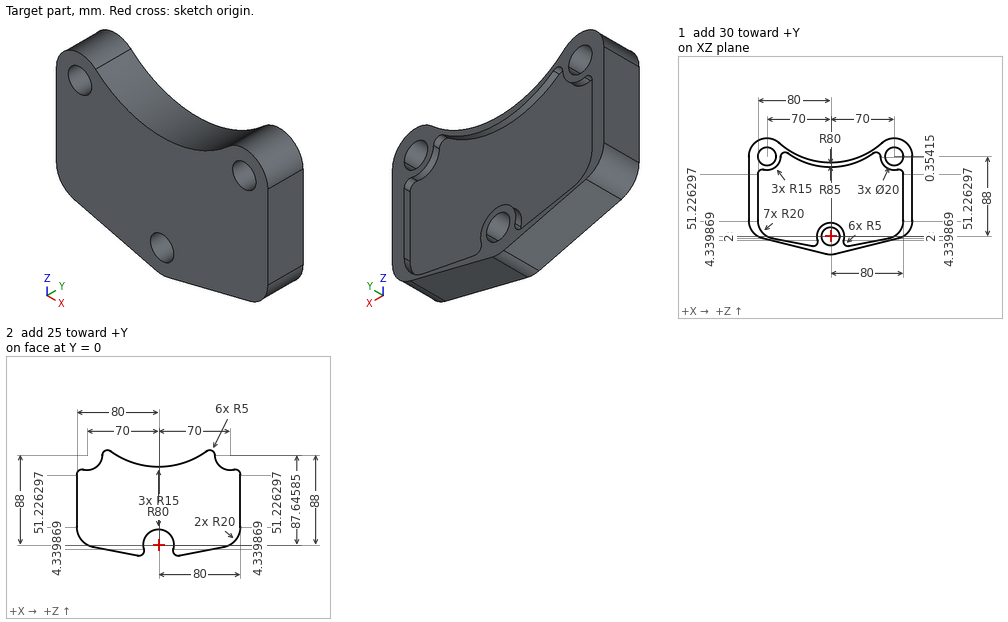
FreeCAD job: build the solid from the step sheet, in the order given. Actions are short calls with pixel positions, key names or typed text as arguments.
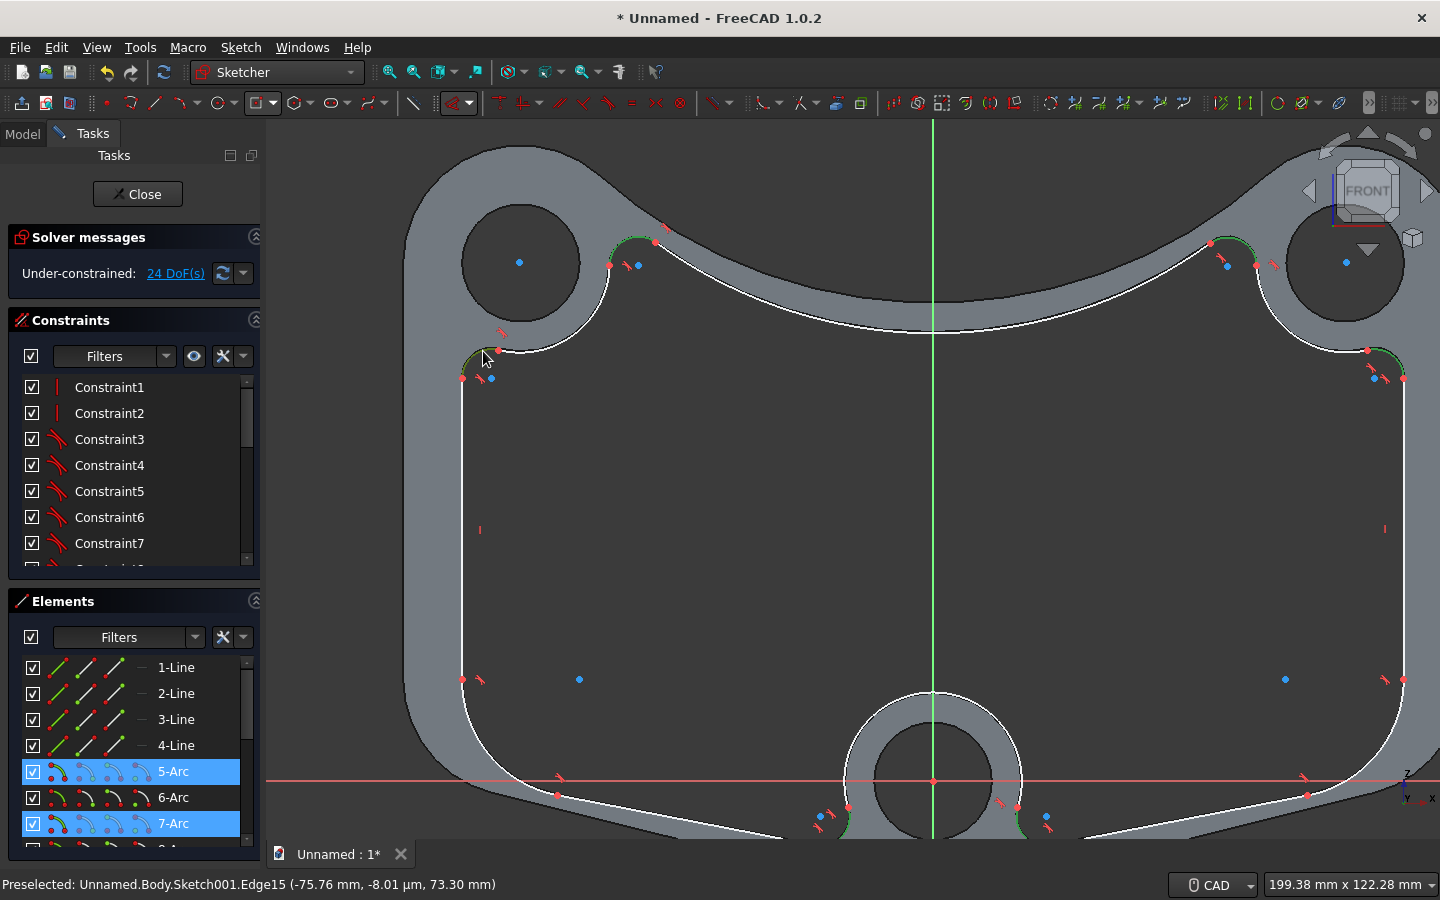
key(e)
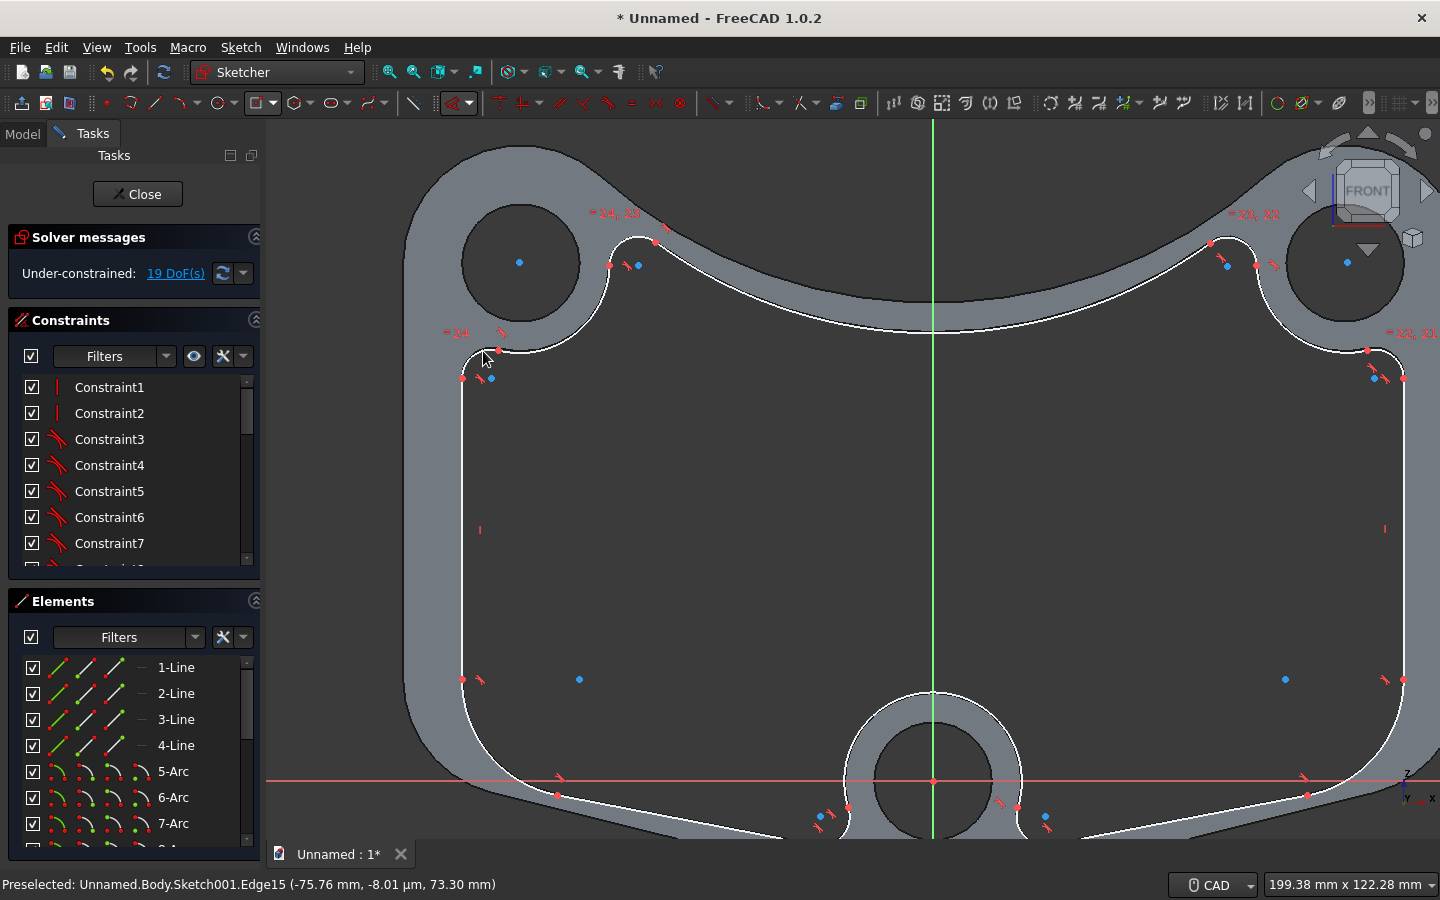
click(993, 716)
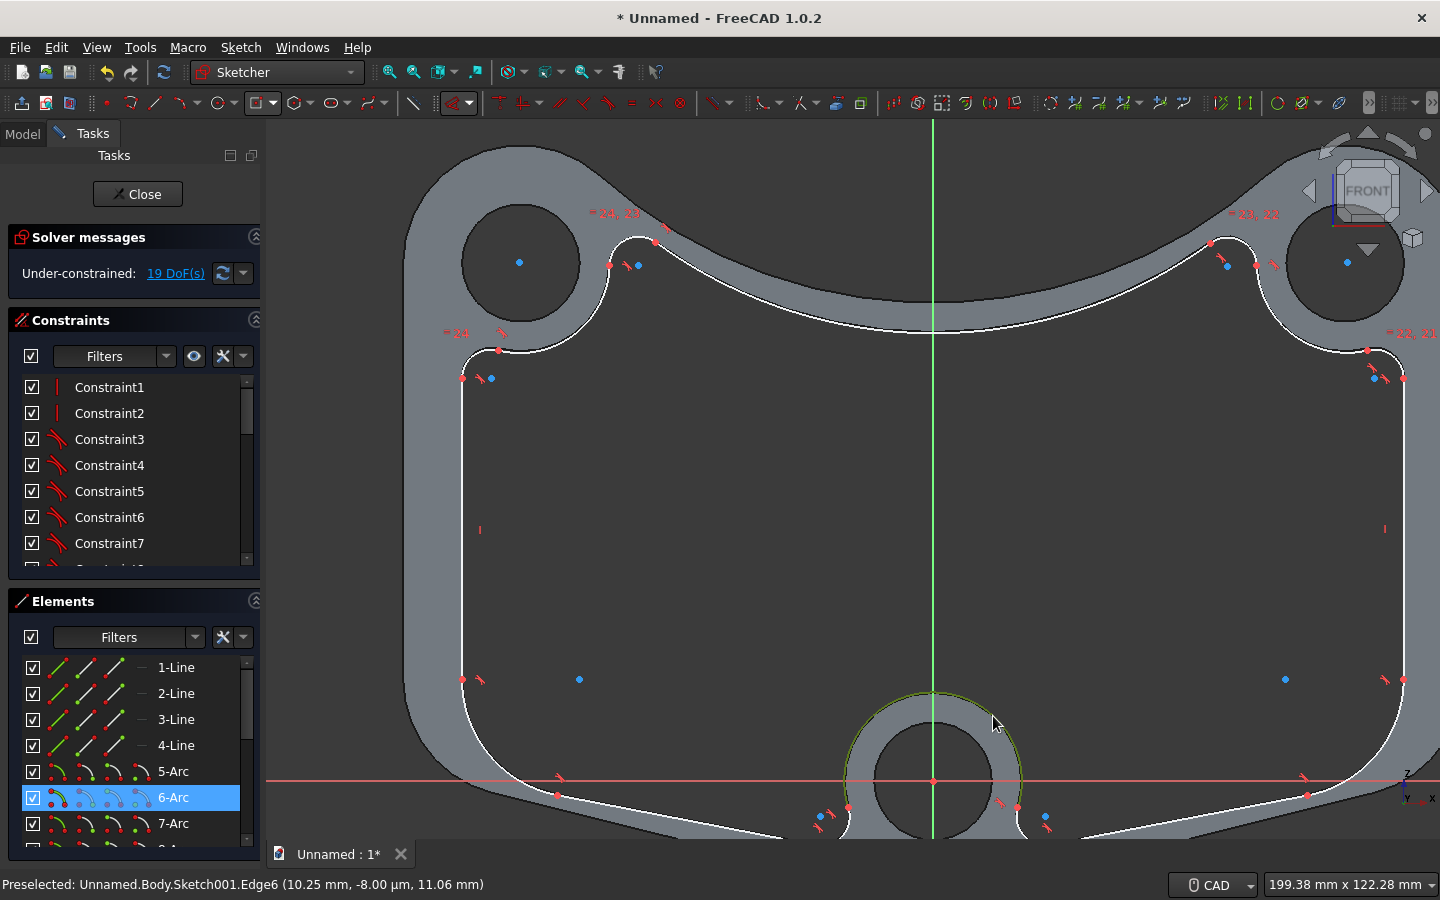
click(1271, 311)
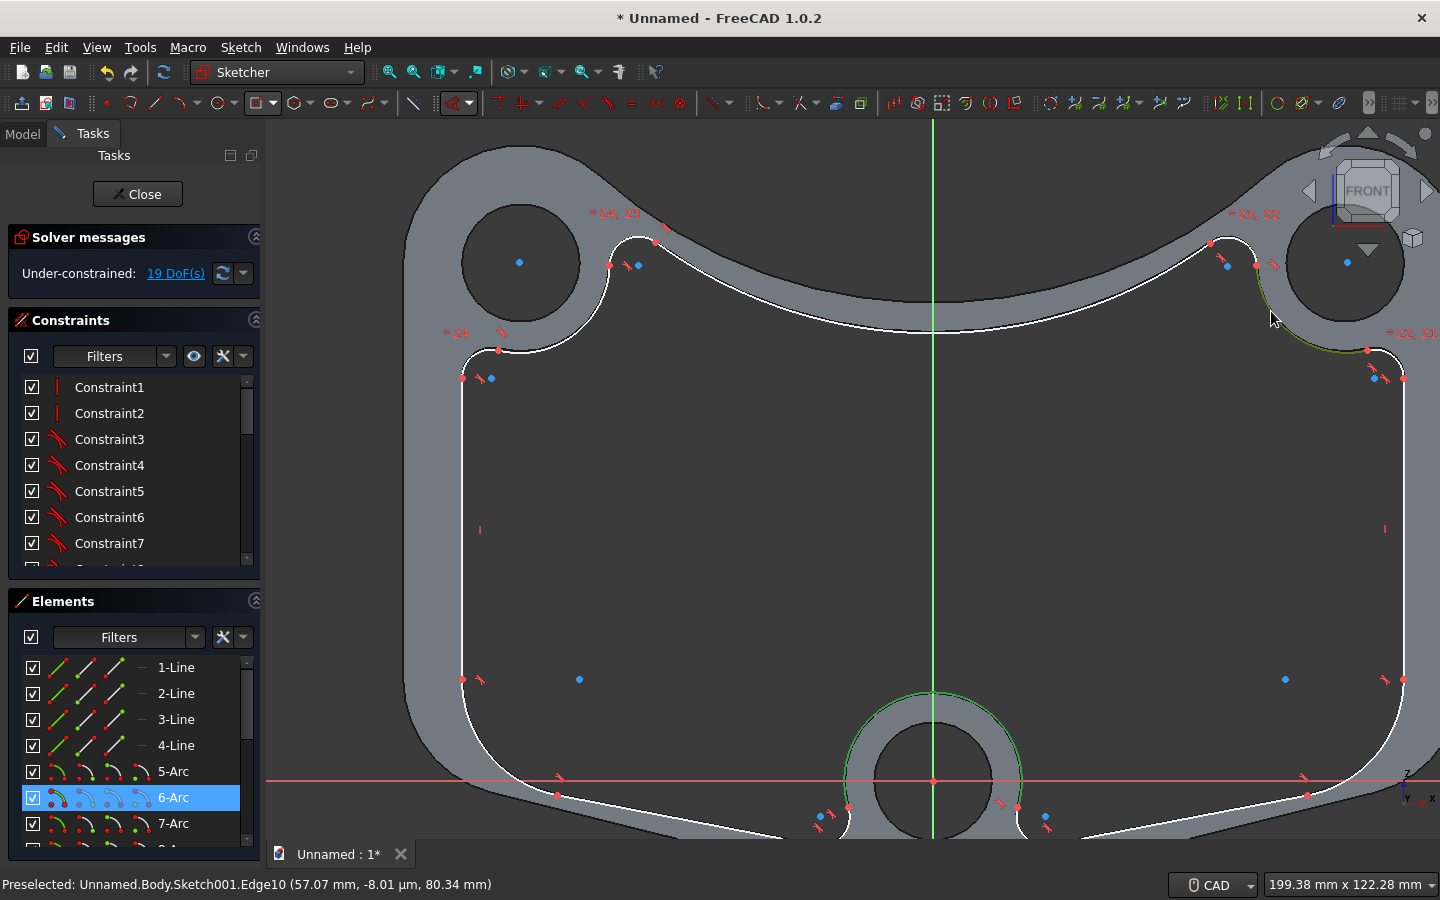
click(546, 349)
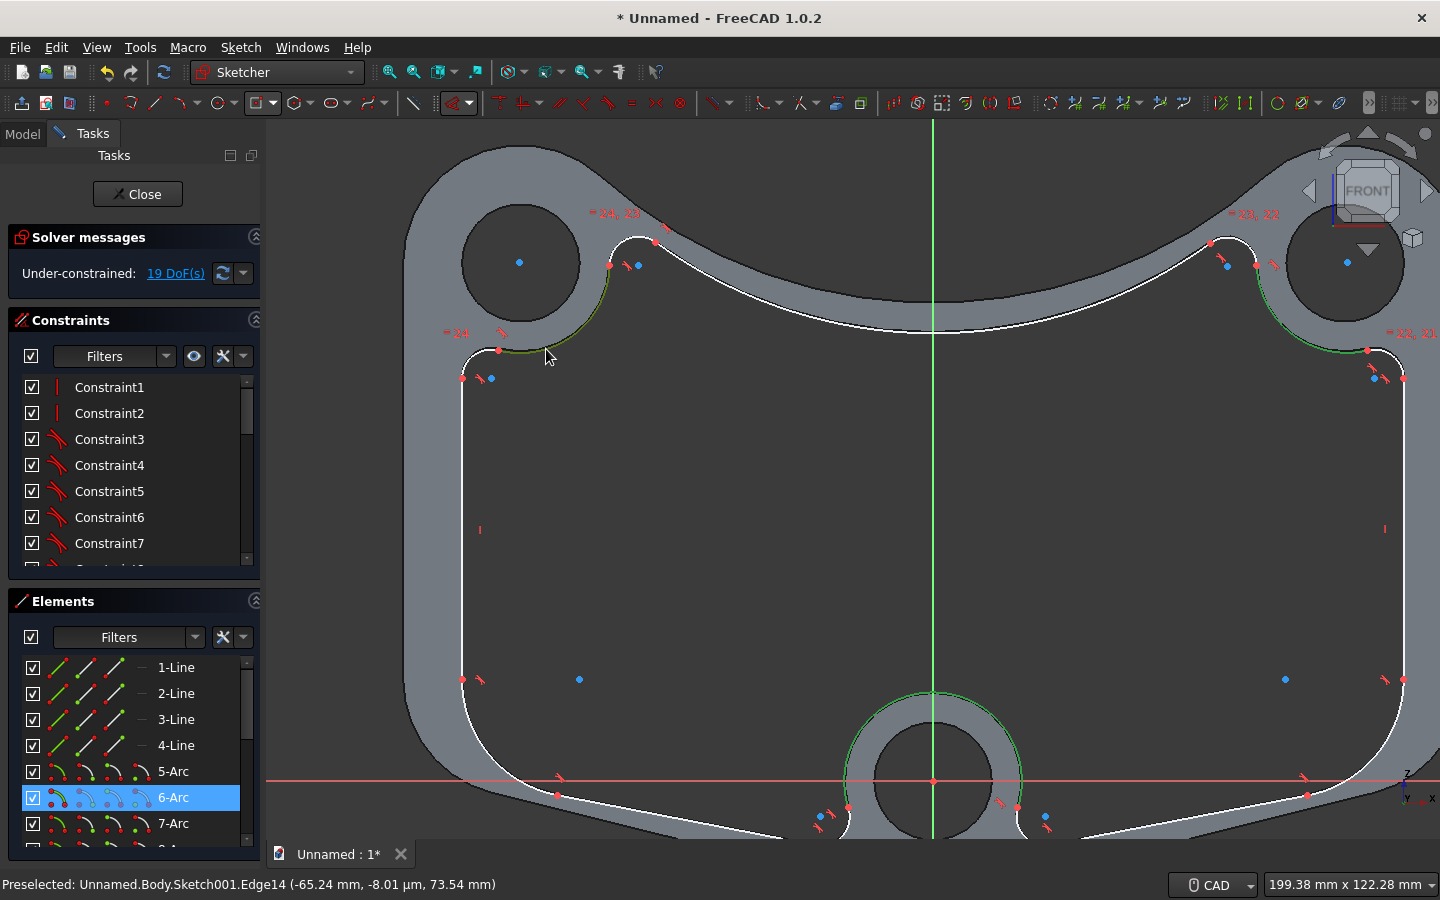
click(632, 104)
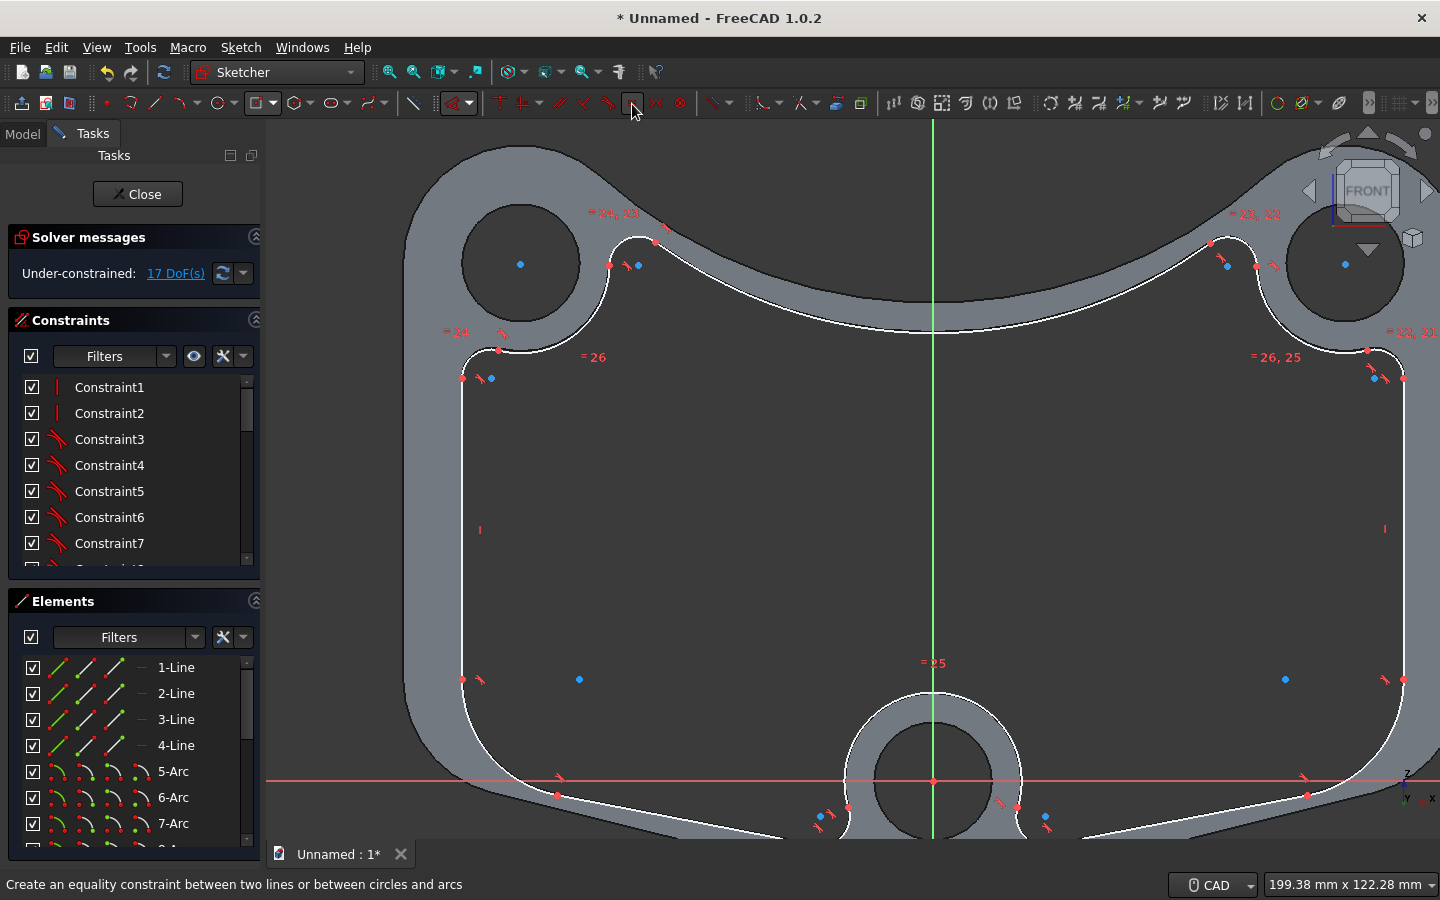
scroll(482, 351, down, 2)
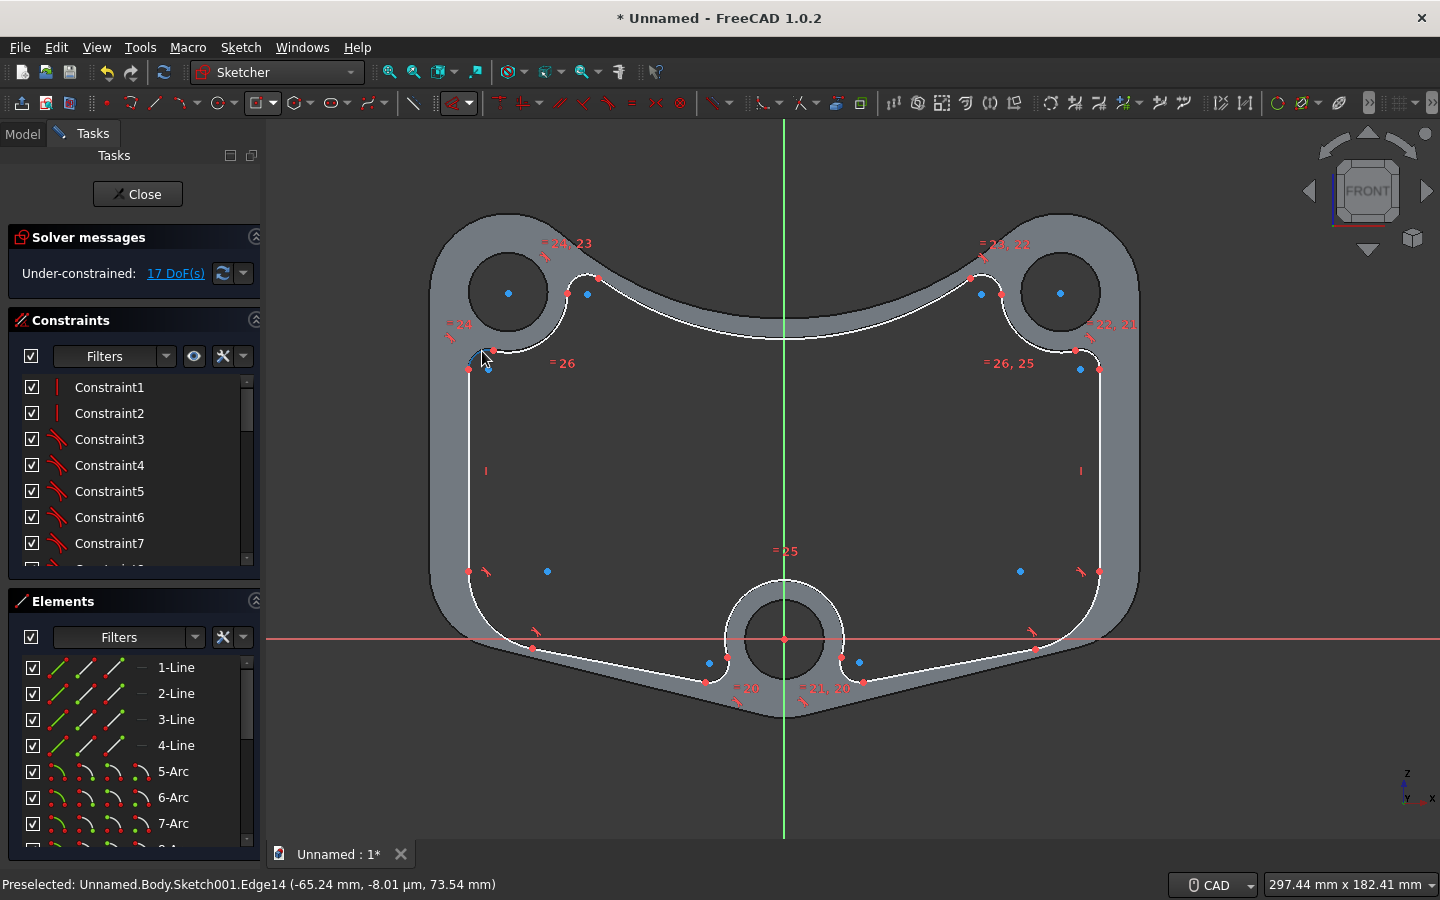
click(1093, 603)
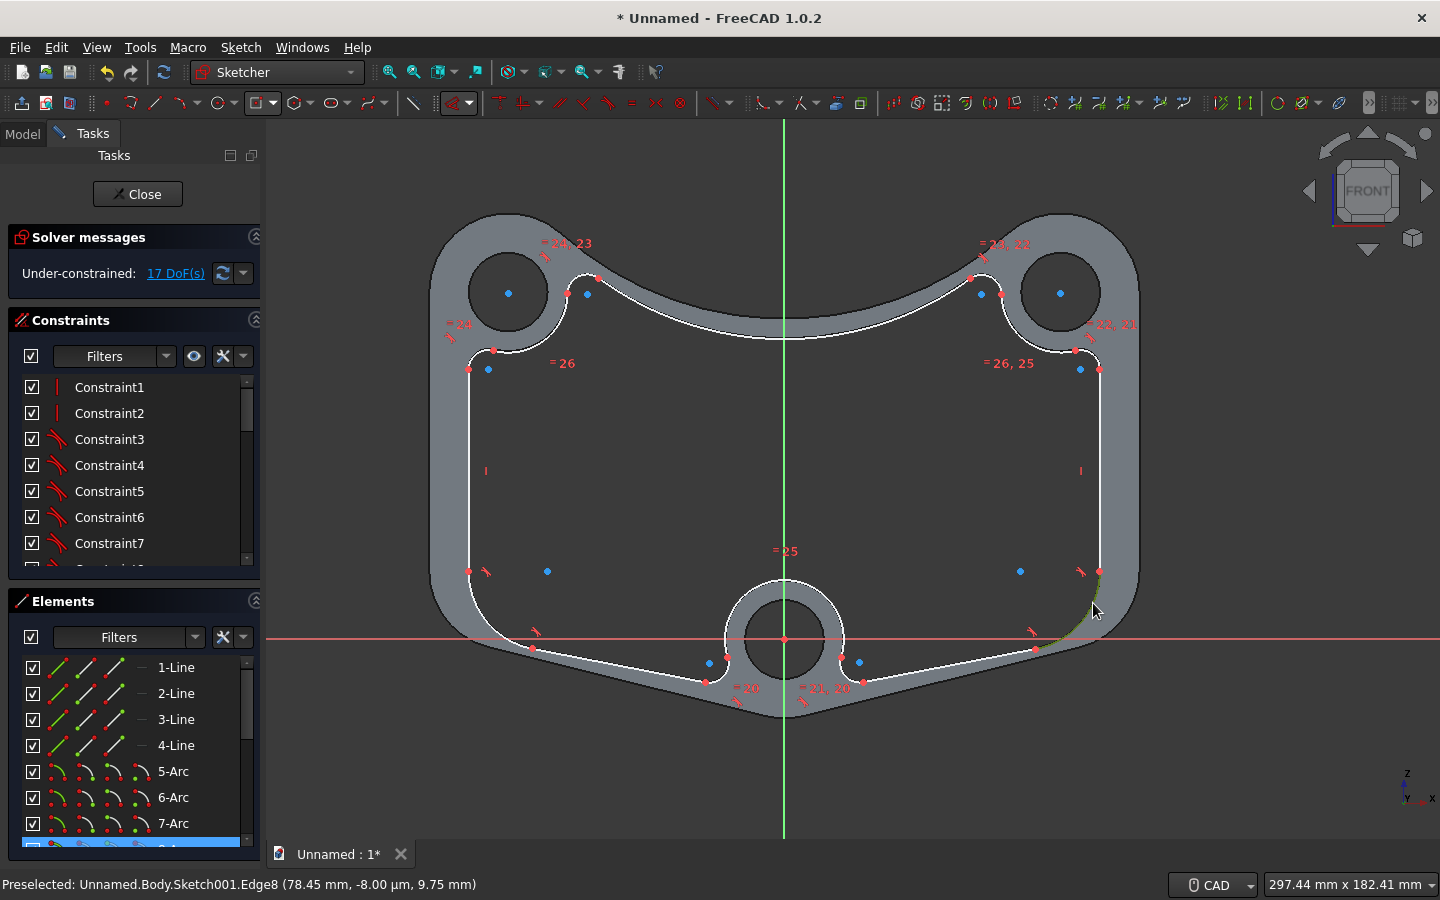
click(475, 603)